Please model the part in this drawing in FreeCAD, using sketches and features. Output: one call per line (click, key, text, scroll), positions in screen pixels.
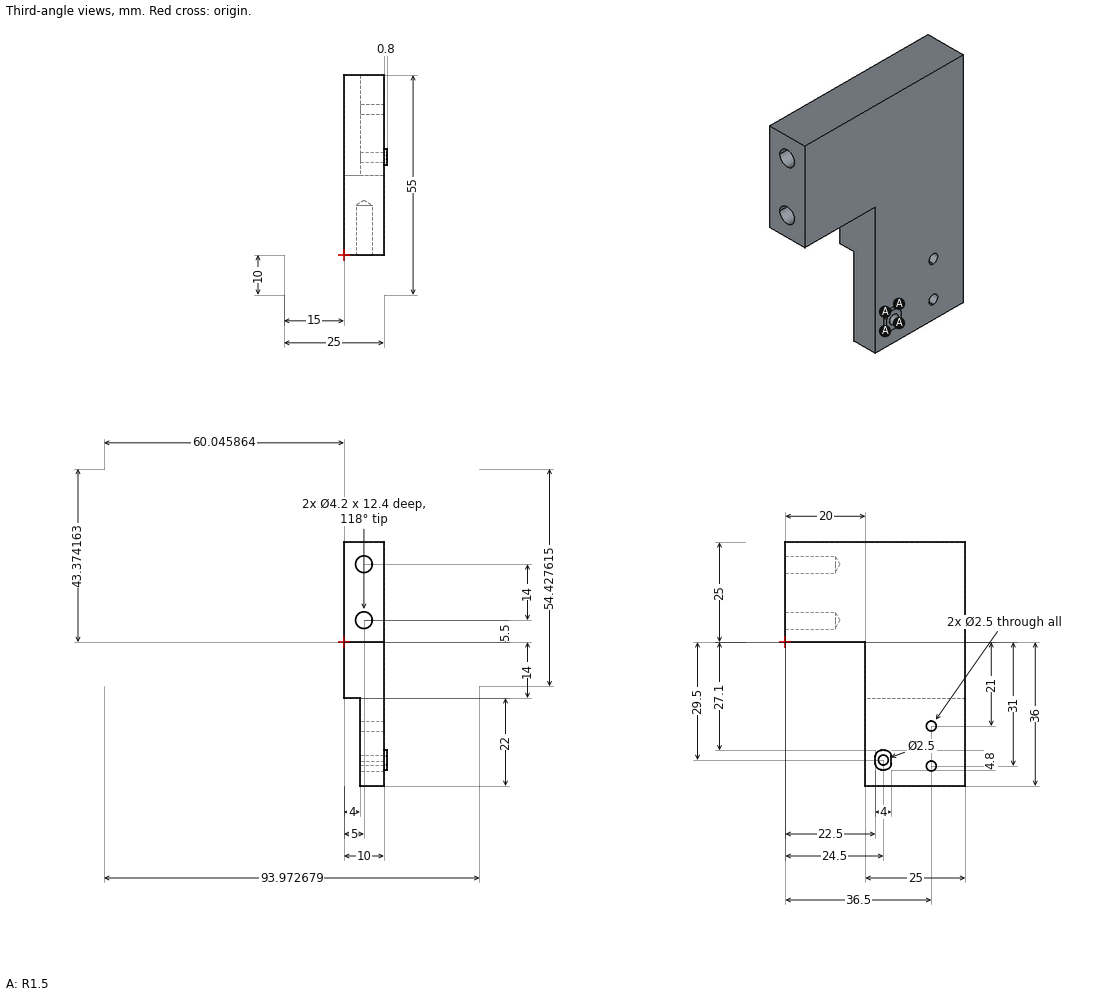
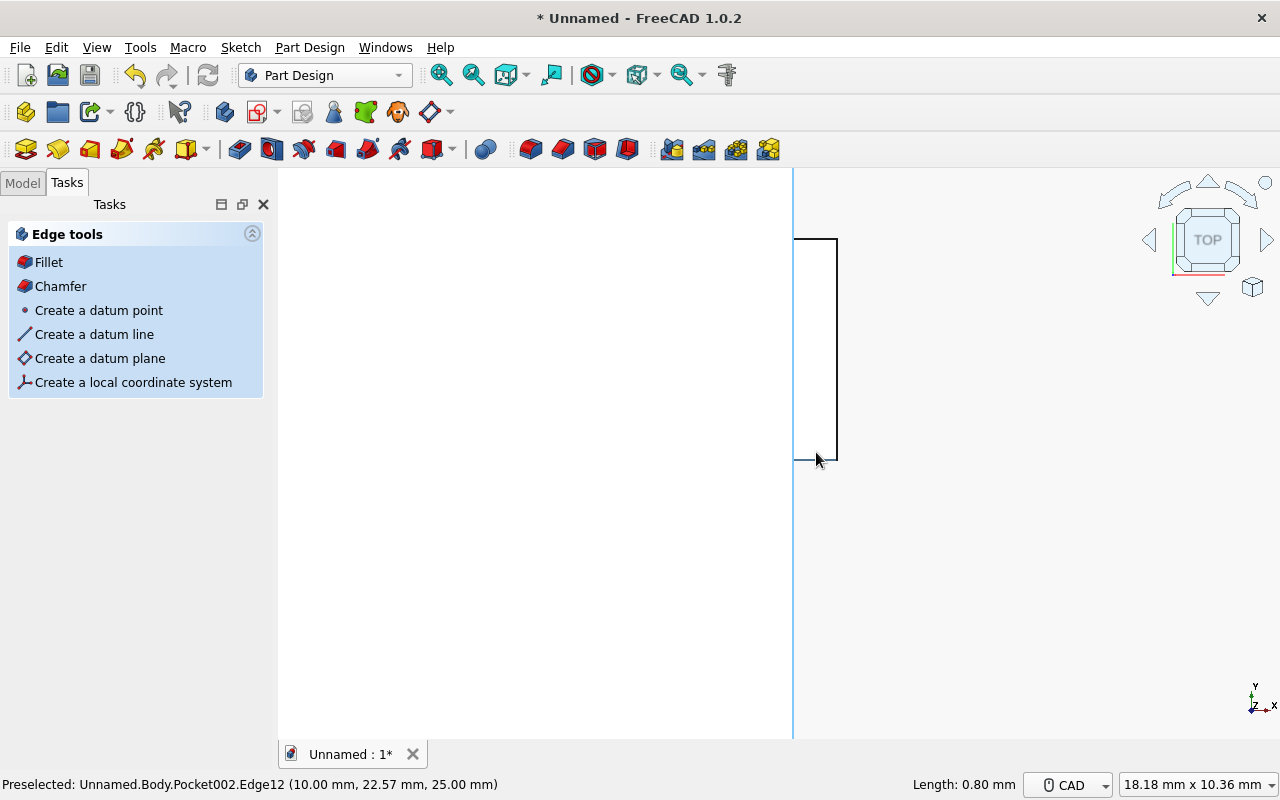
click(815, 238, ctrl)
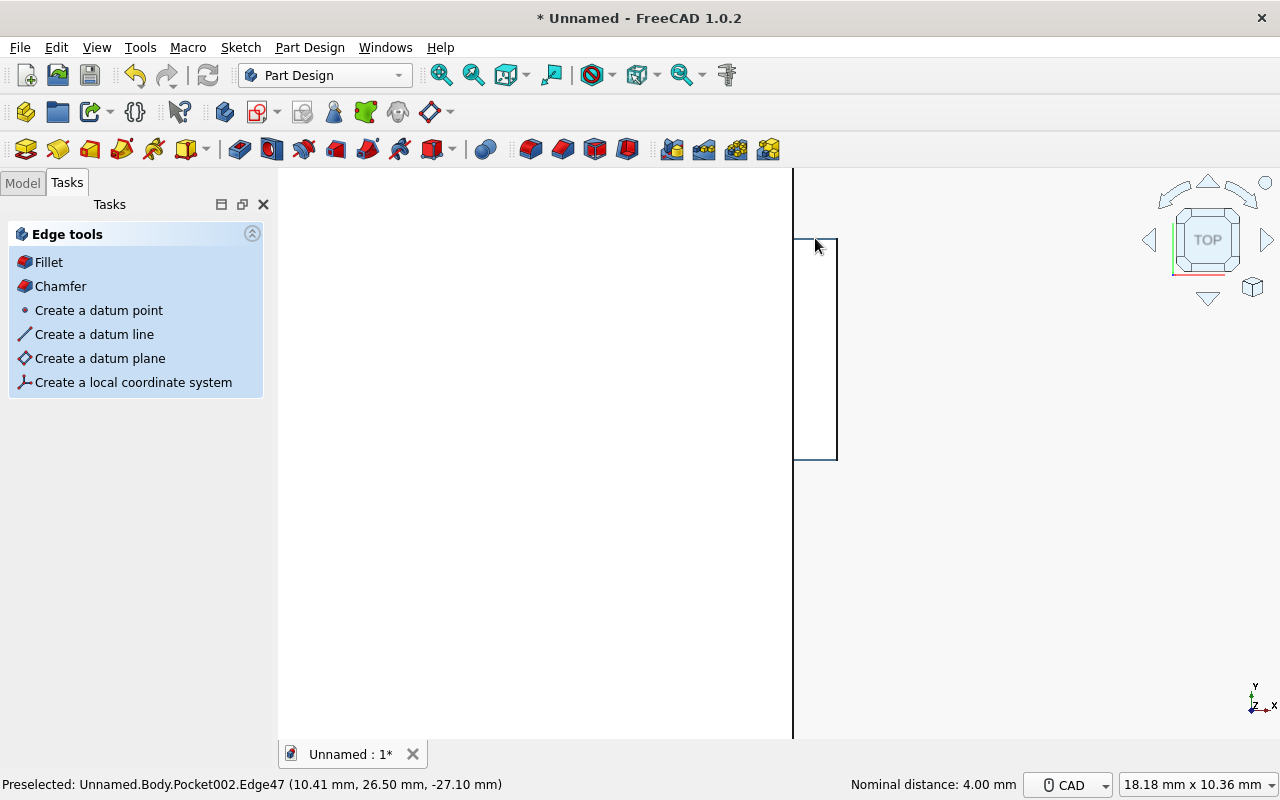
click(442, 76)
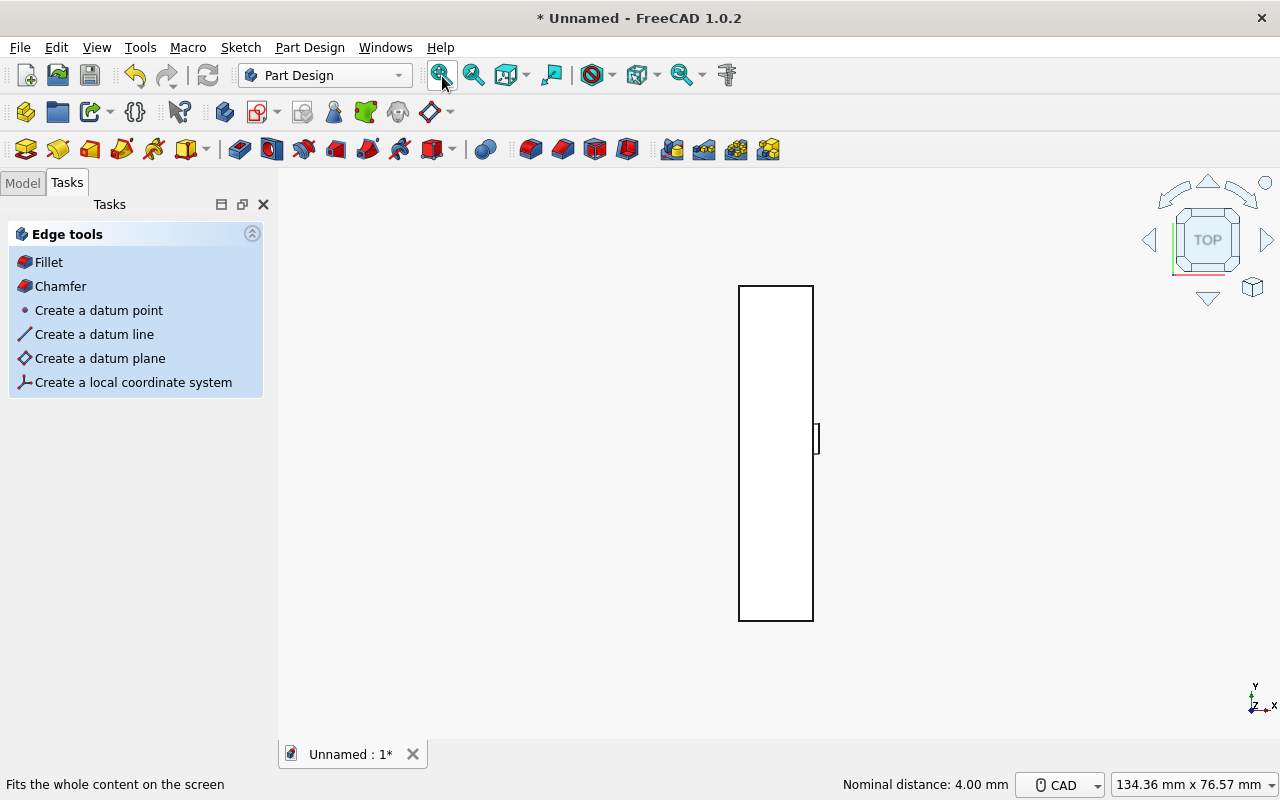
key(1)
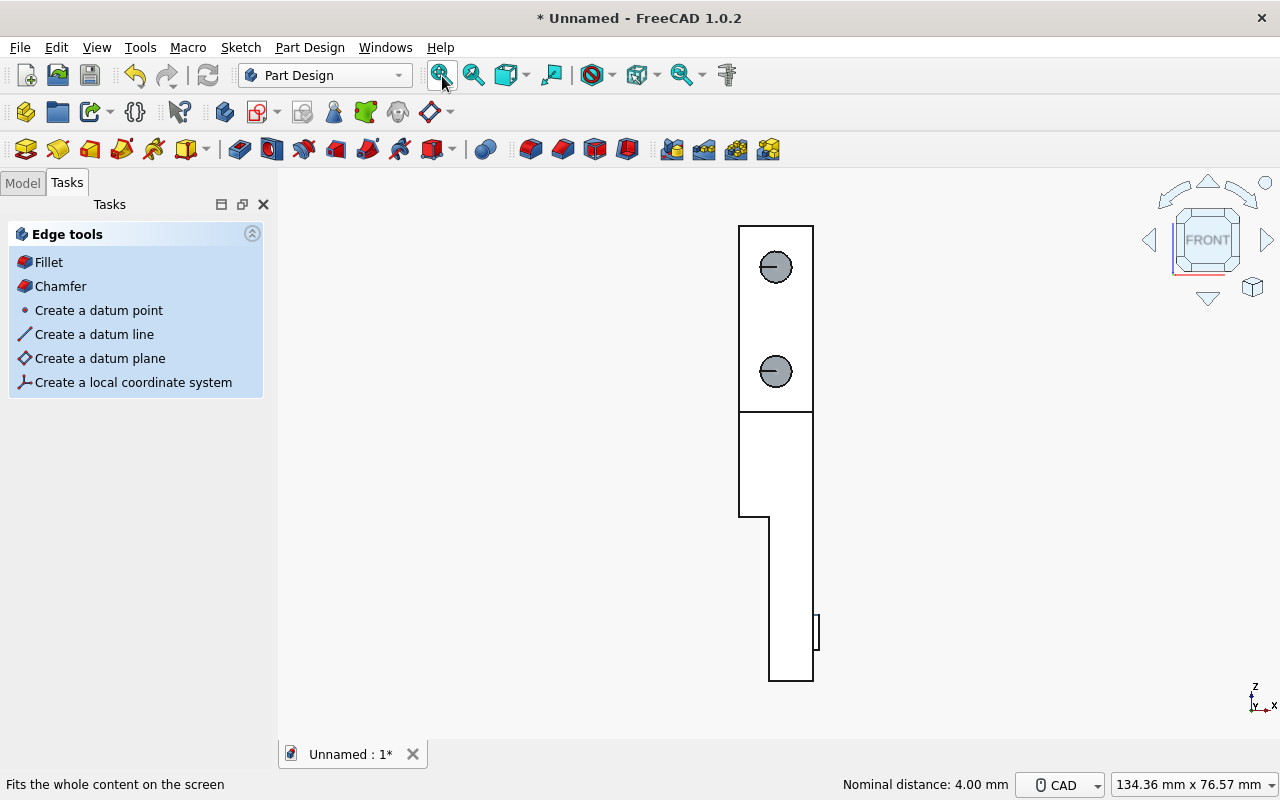
scroll(816, 649, up, 10)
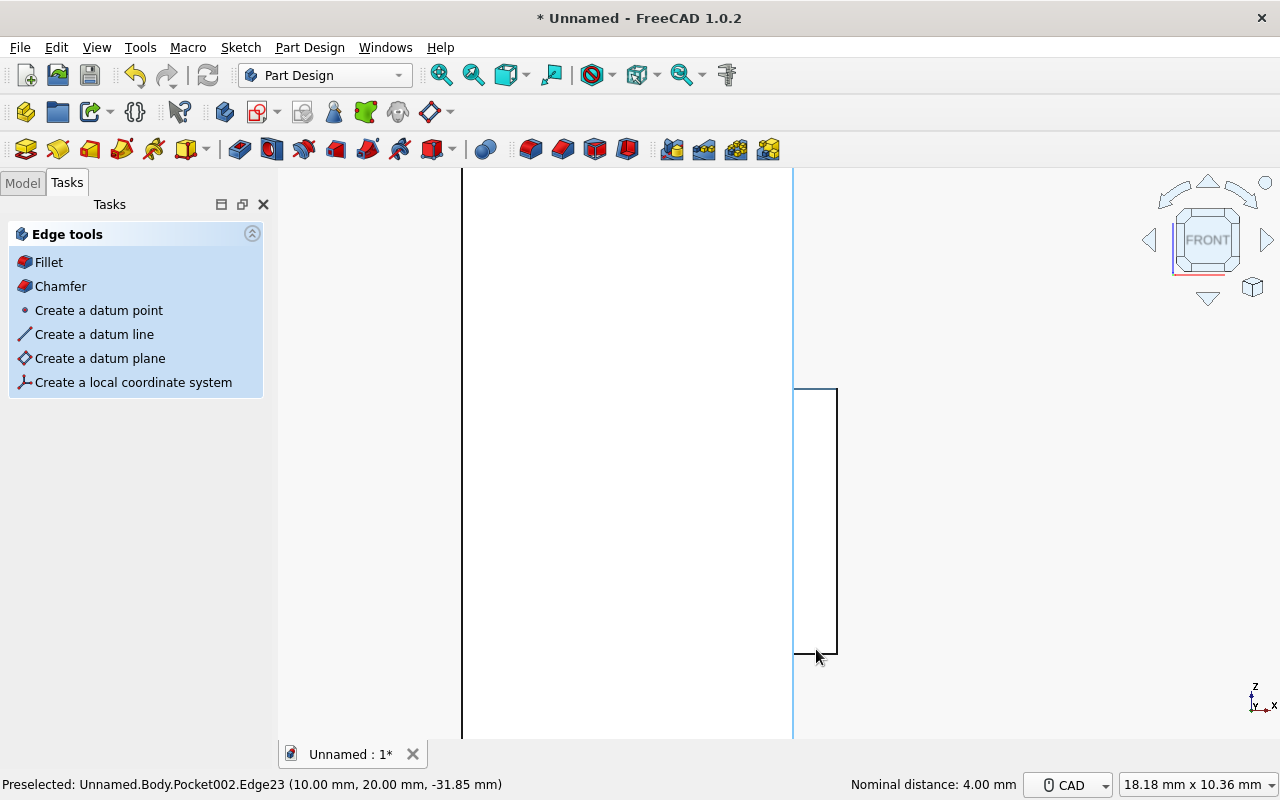
click(815, 653, ctrl)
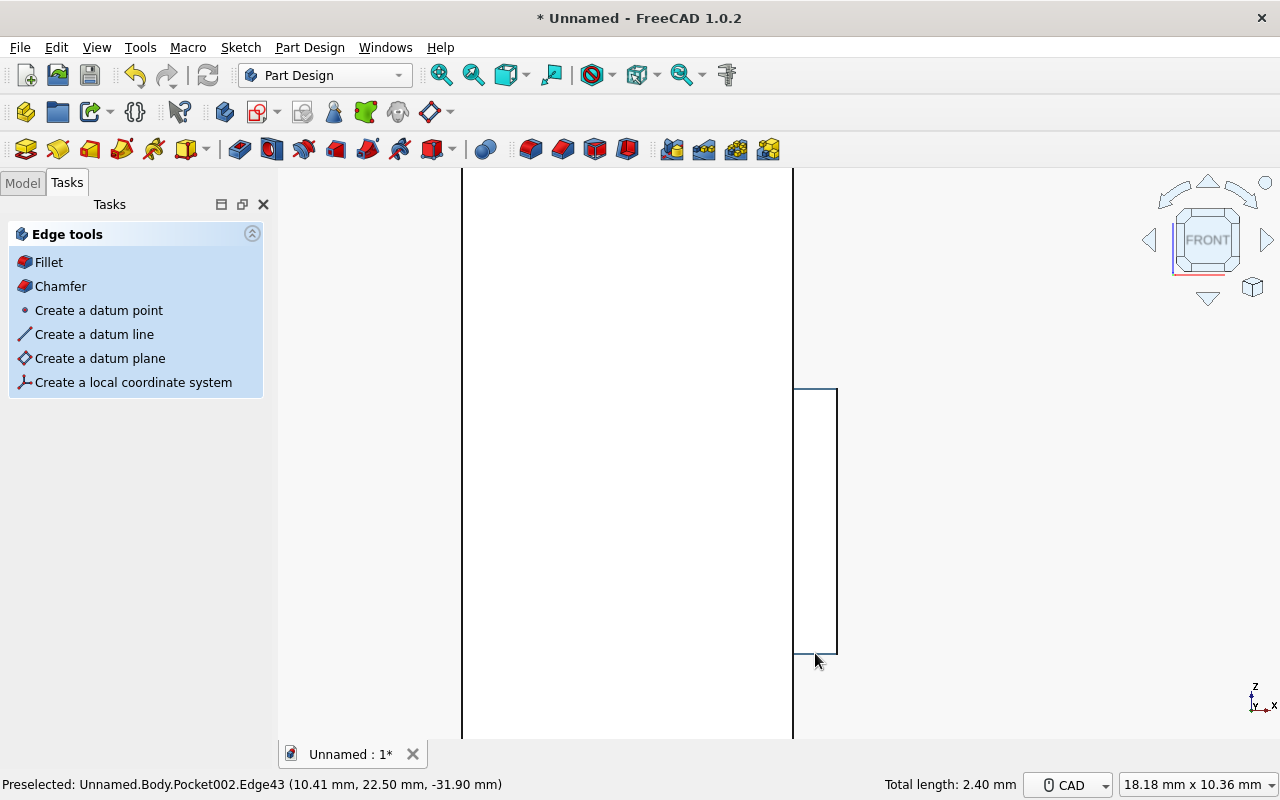
key(v)
key(f)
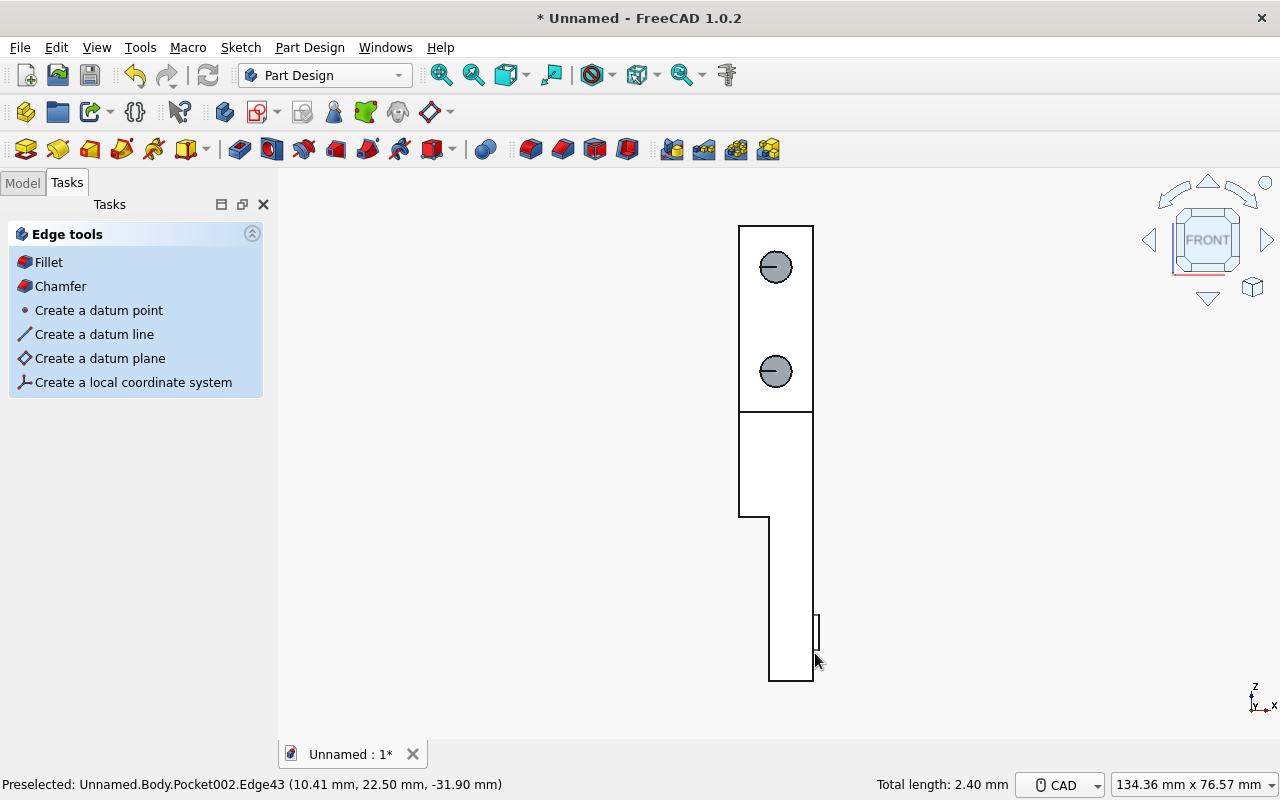
key(3)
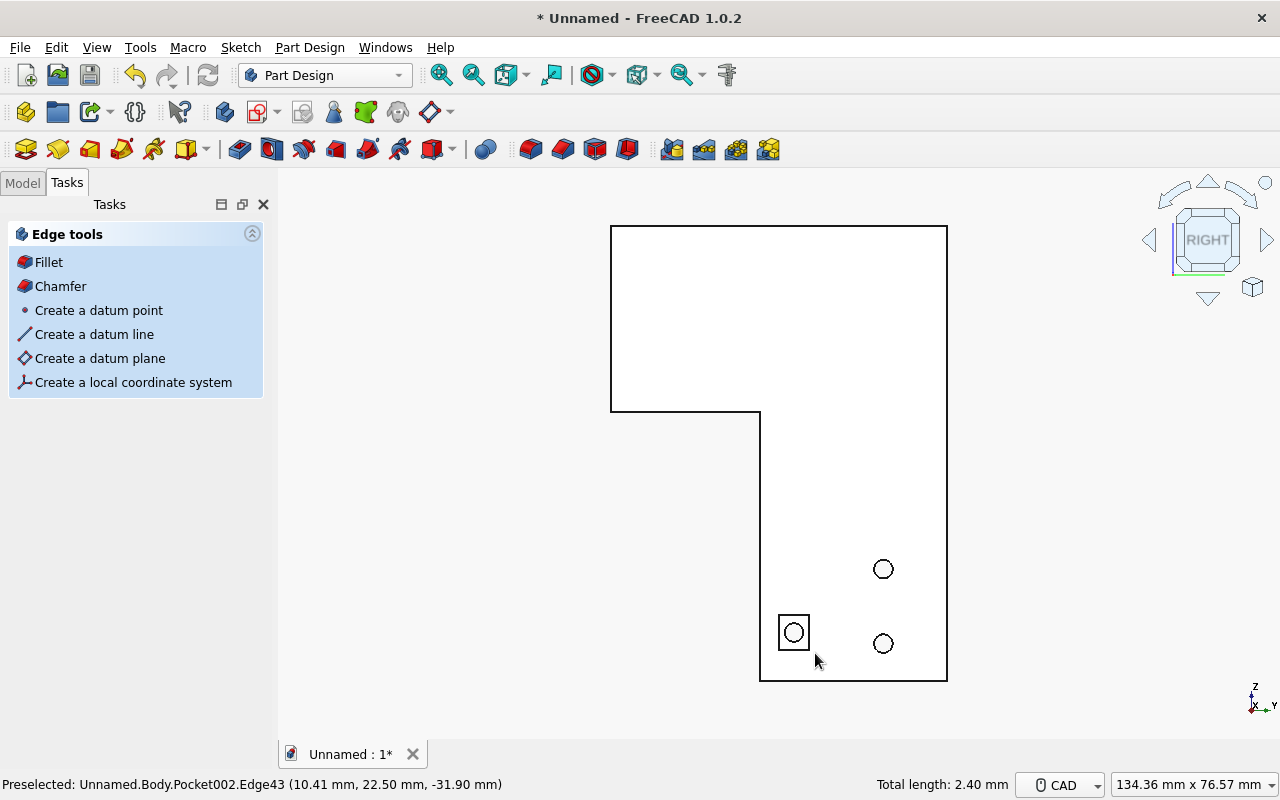
scroll(809, 649, up, 10)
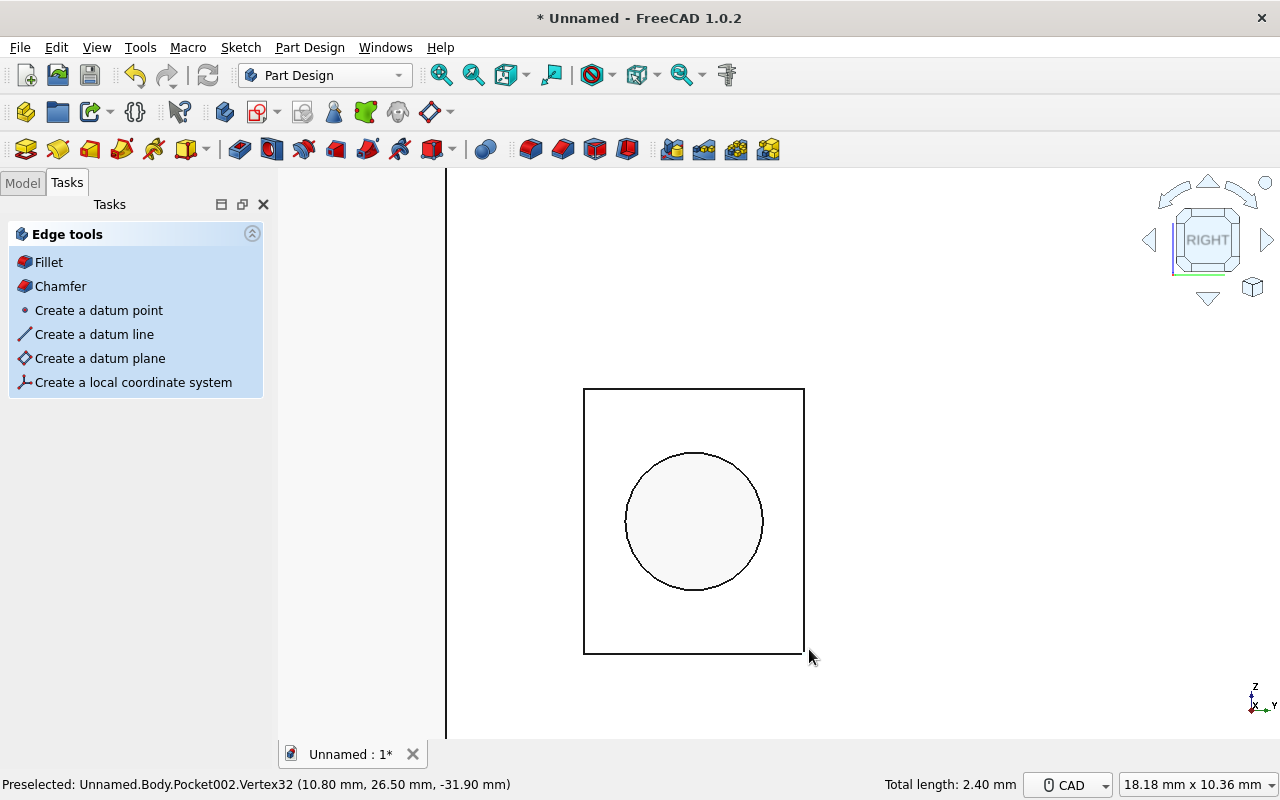
click(442, 76)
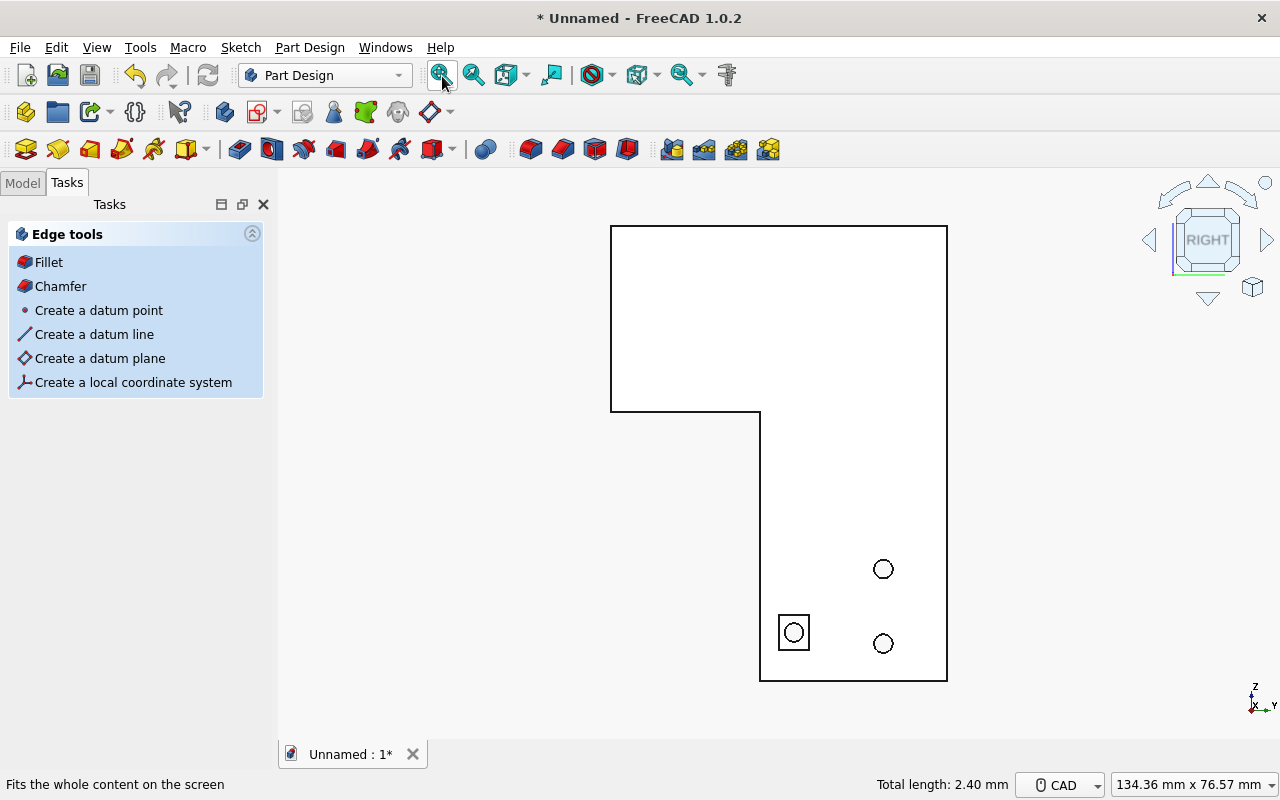
key(5)